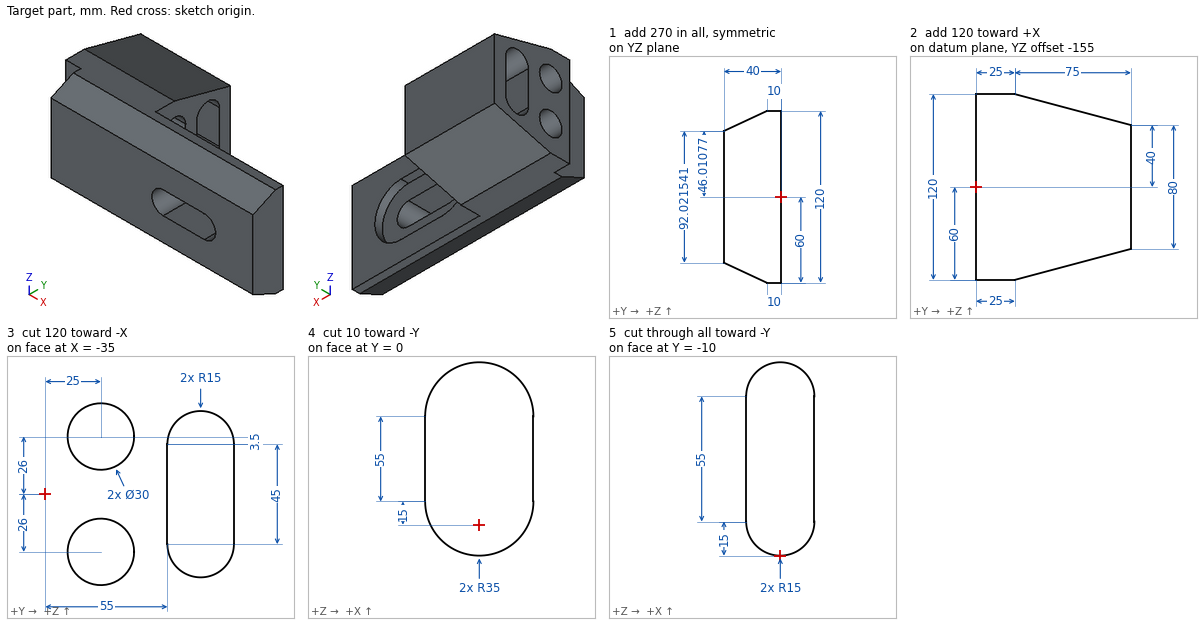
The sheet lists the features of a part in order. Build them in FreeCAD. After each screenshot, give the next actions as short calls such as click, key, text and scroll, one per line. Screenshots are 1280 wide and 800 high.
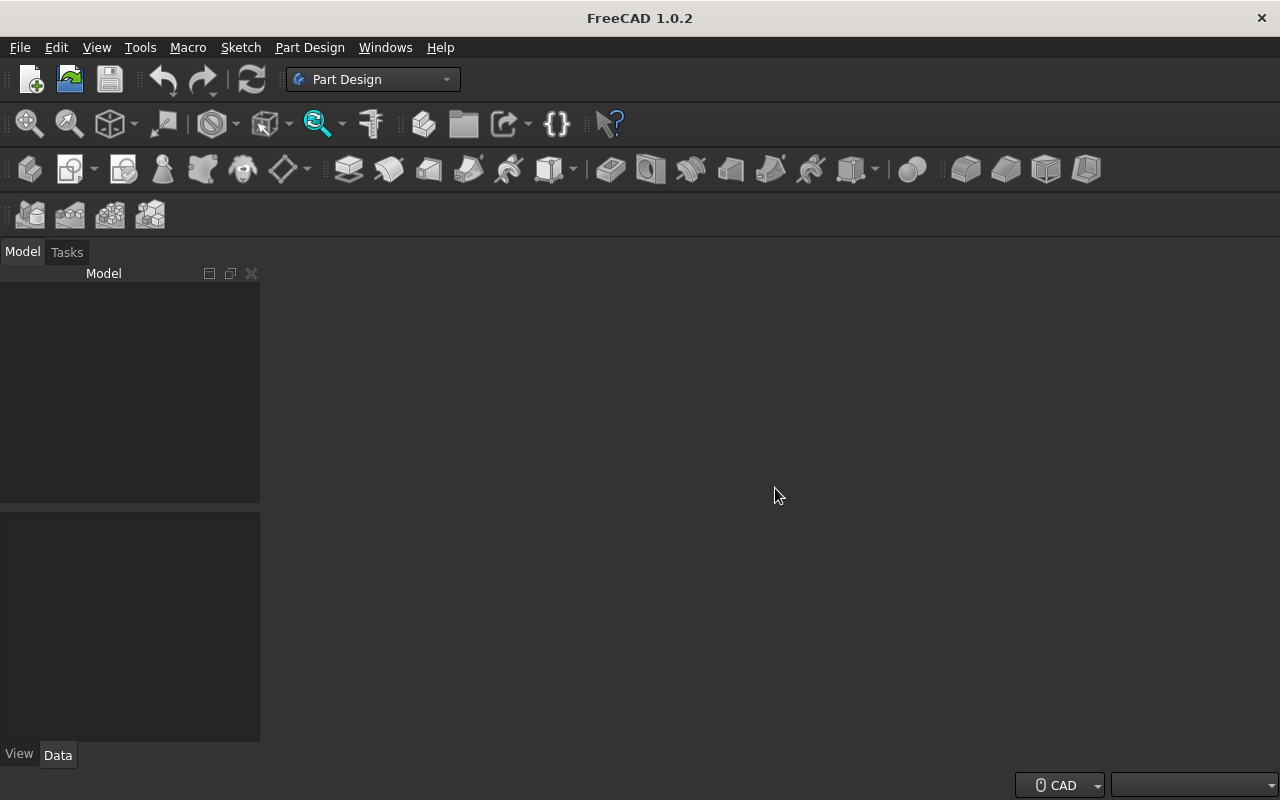
click(30, 80)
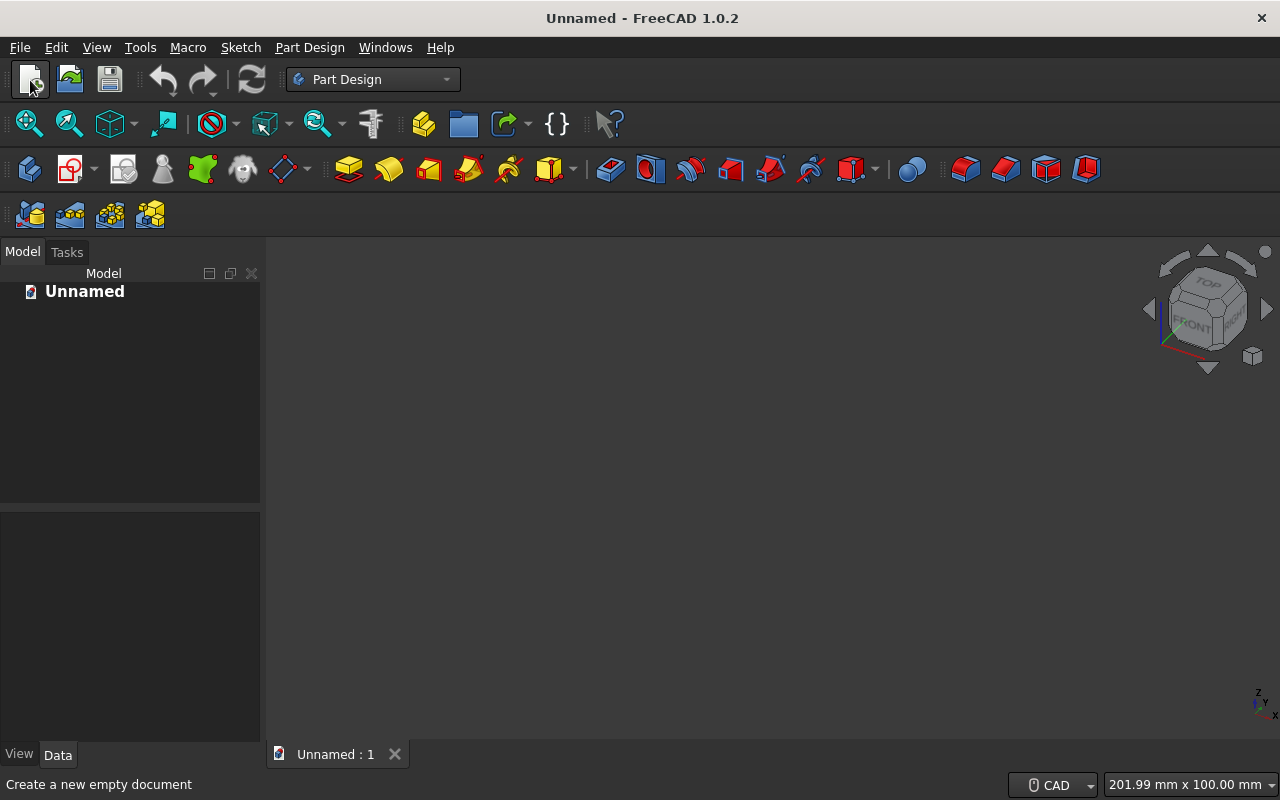
click(70, 170)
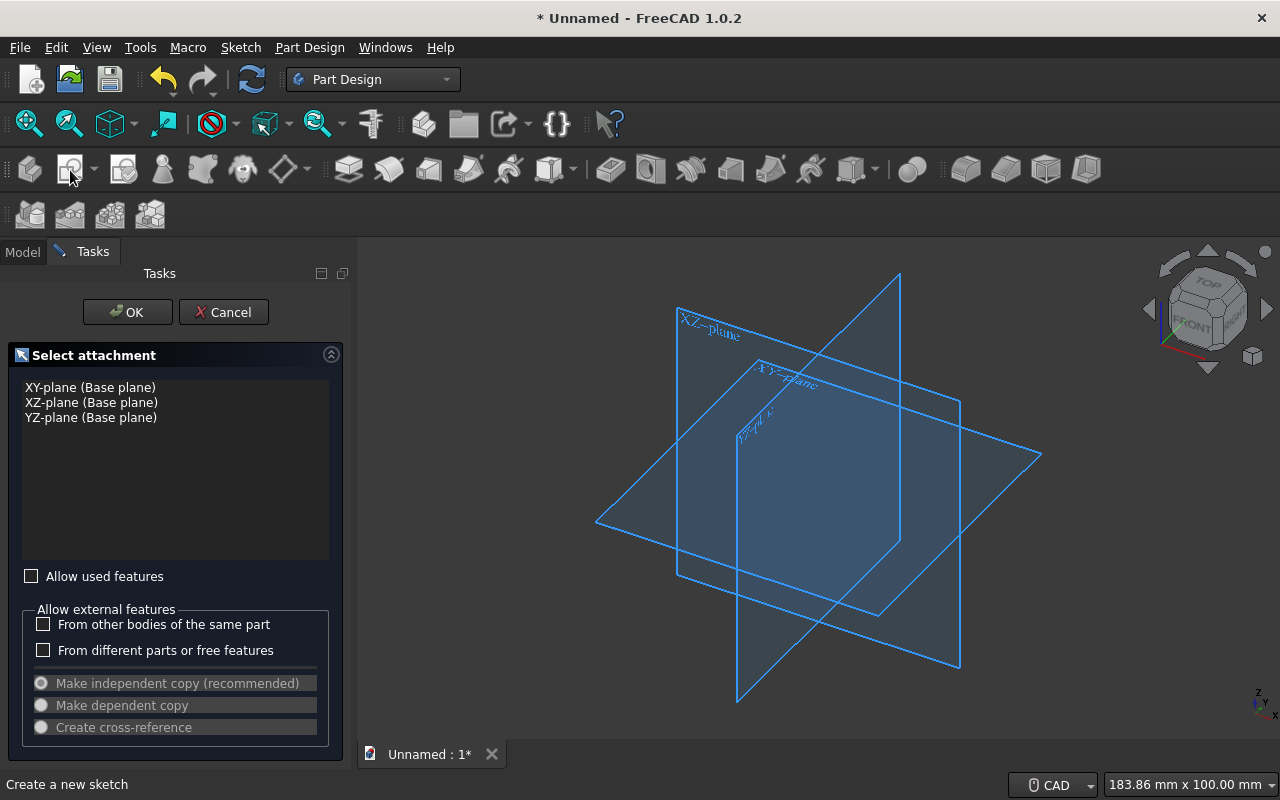
click(82, 418)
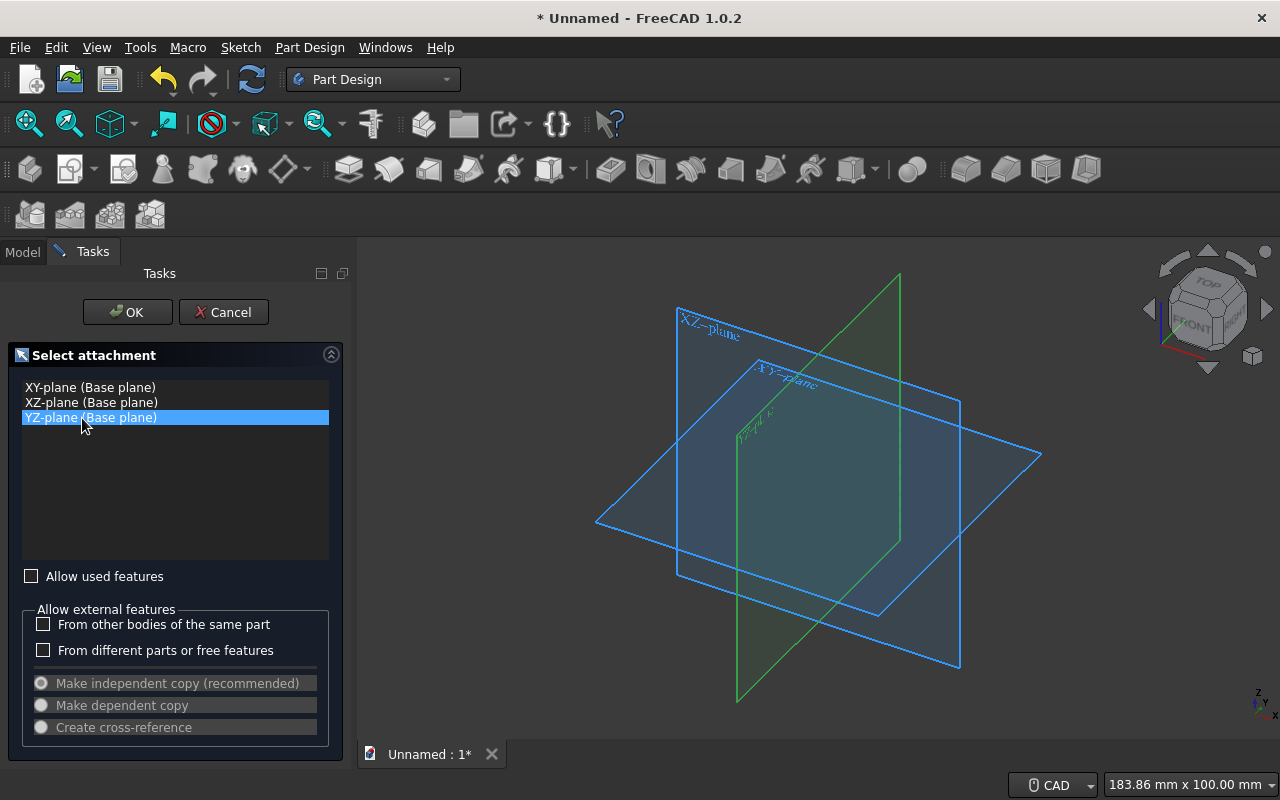
click(128, 312)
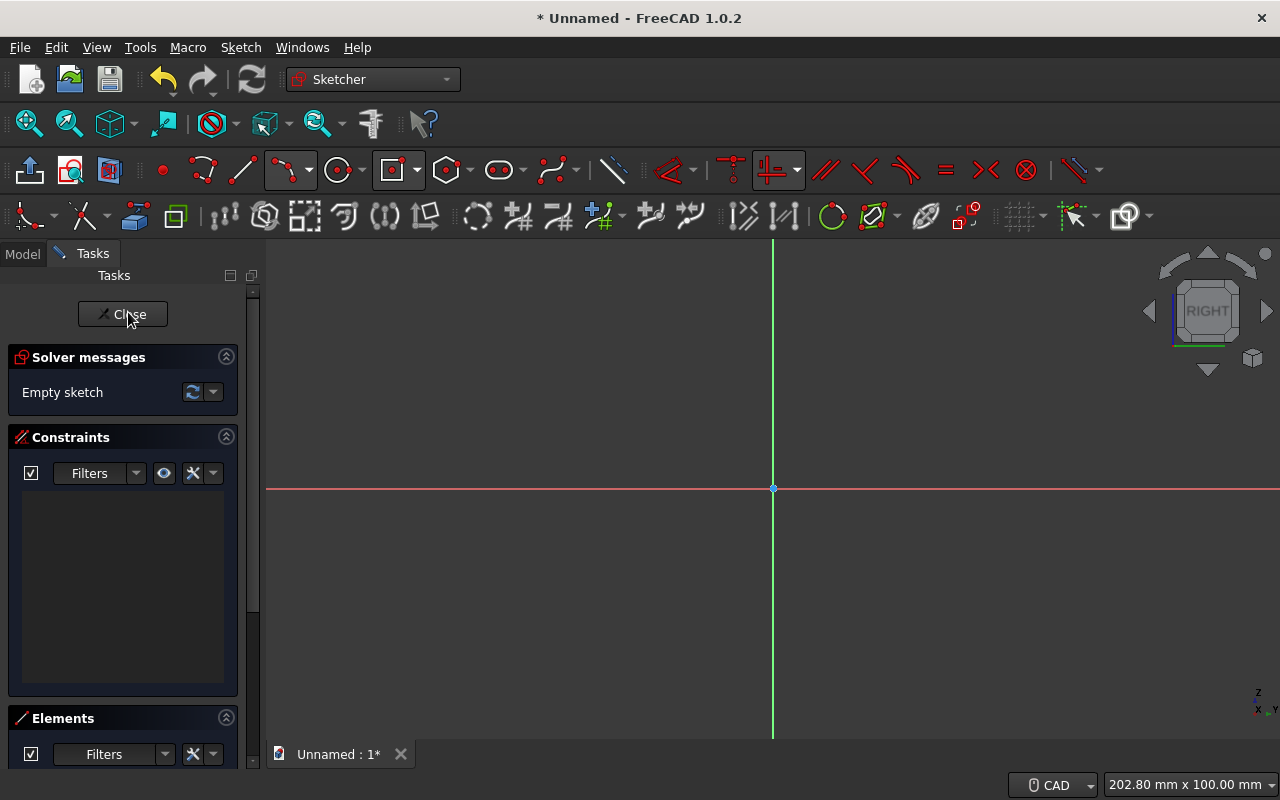
scroll(743, 489, down, 3)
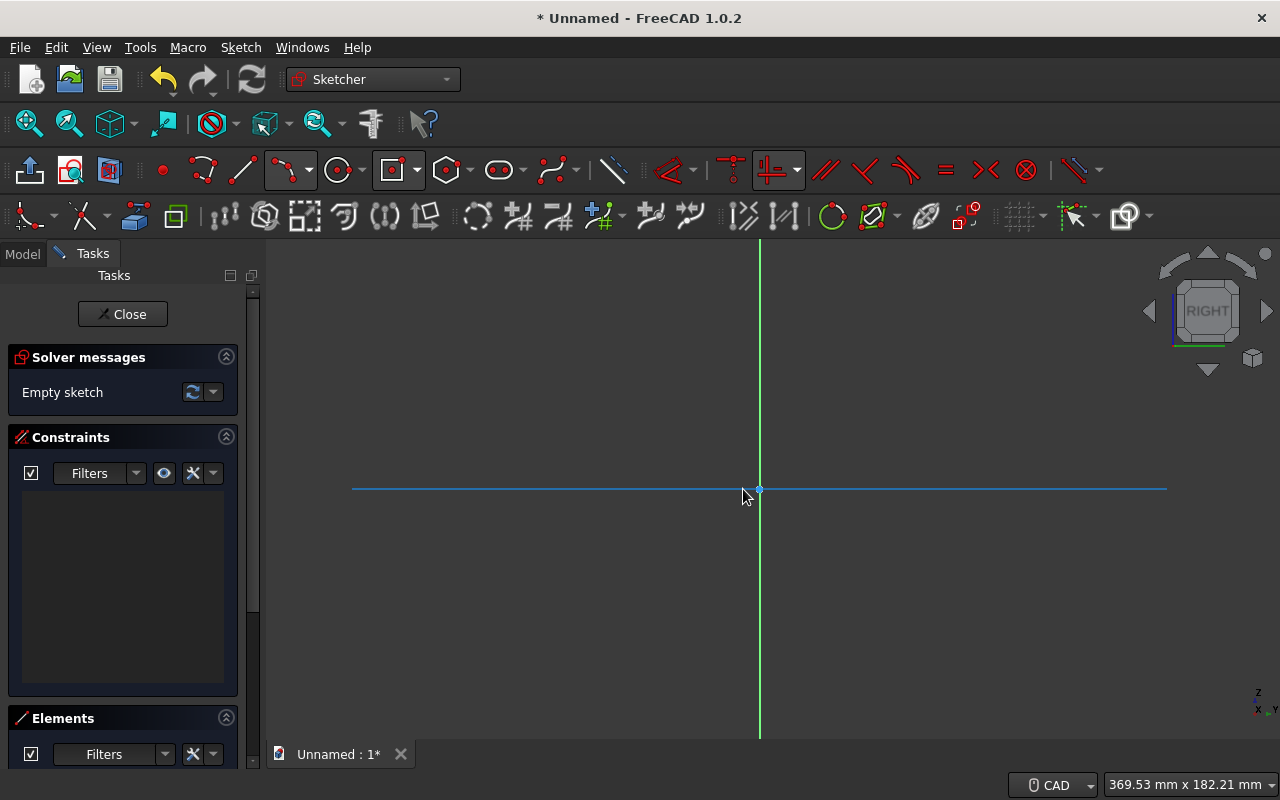
click(204, 170)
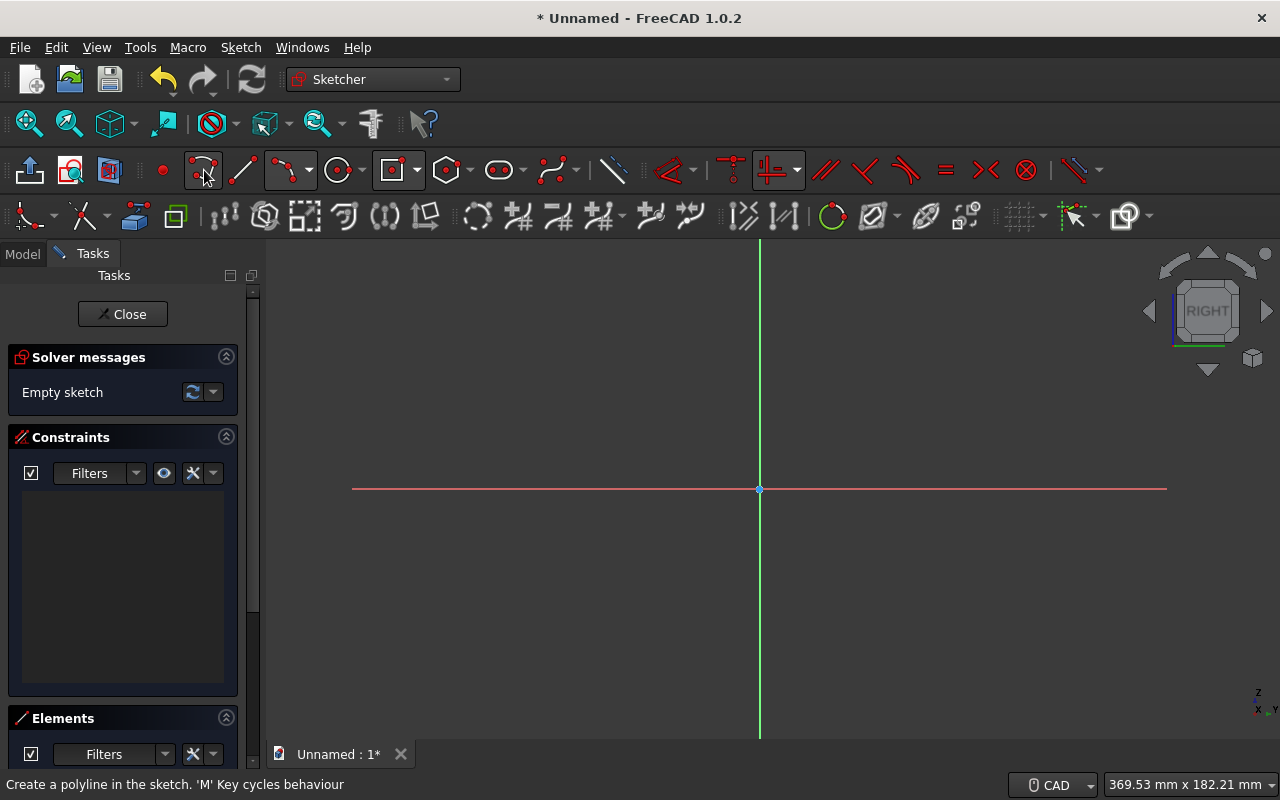
click(760, 654)
click(751, 325)
click(732, 325)
click(650, 363)
click(650, 615)
click(732, 654)
click(760, 655)
key(Escape)
key(Escape)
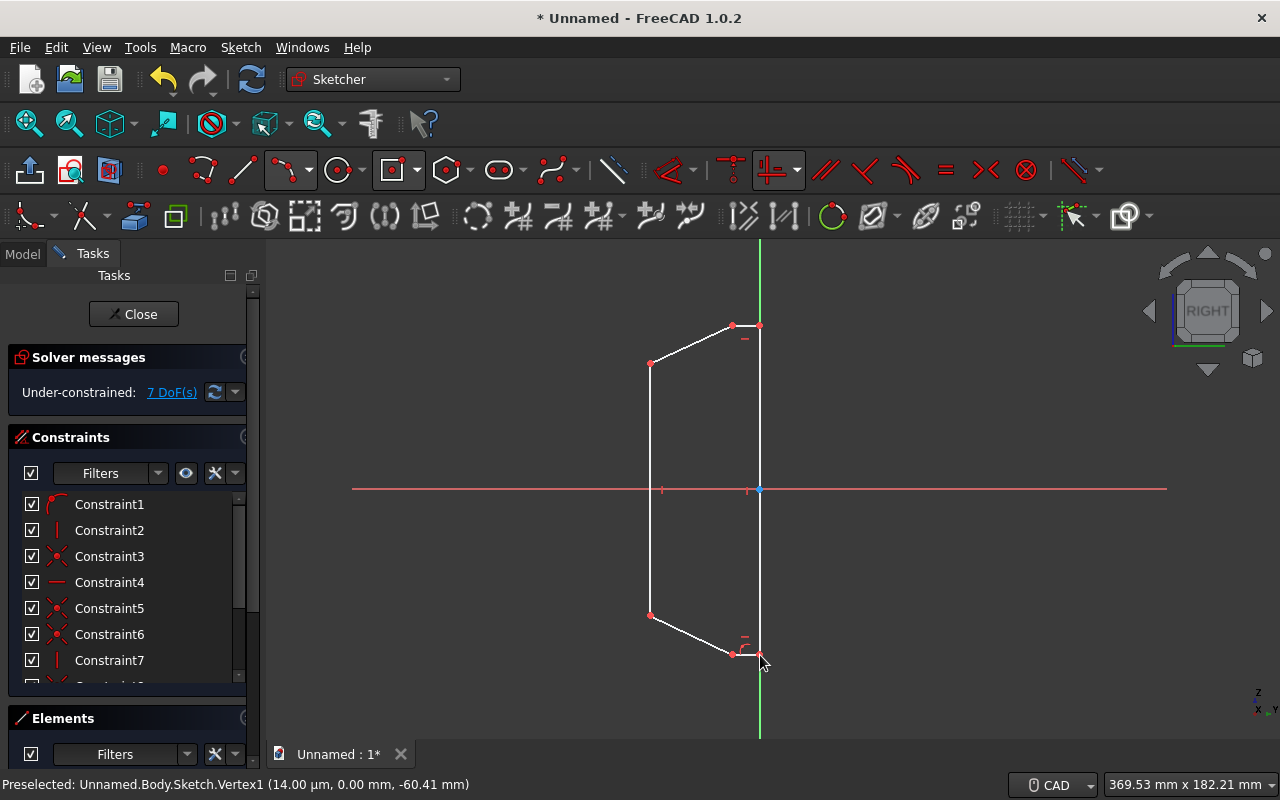
click(668, 170)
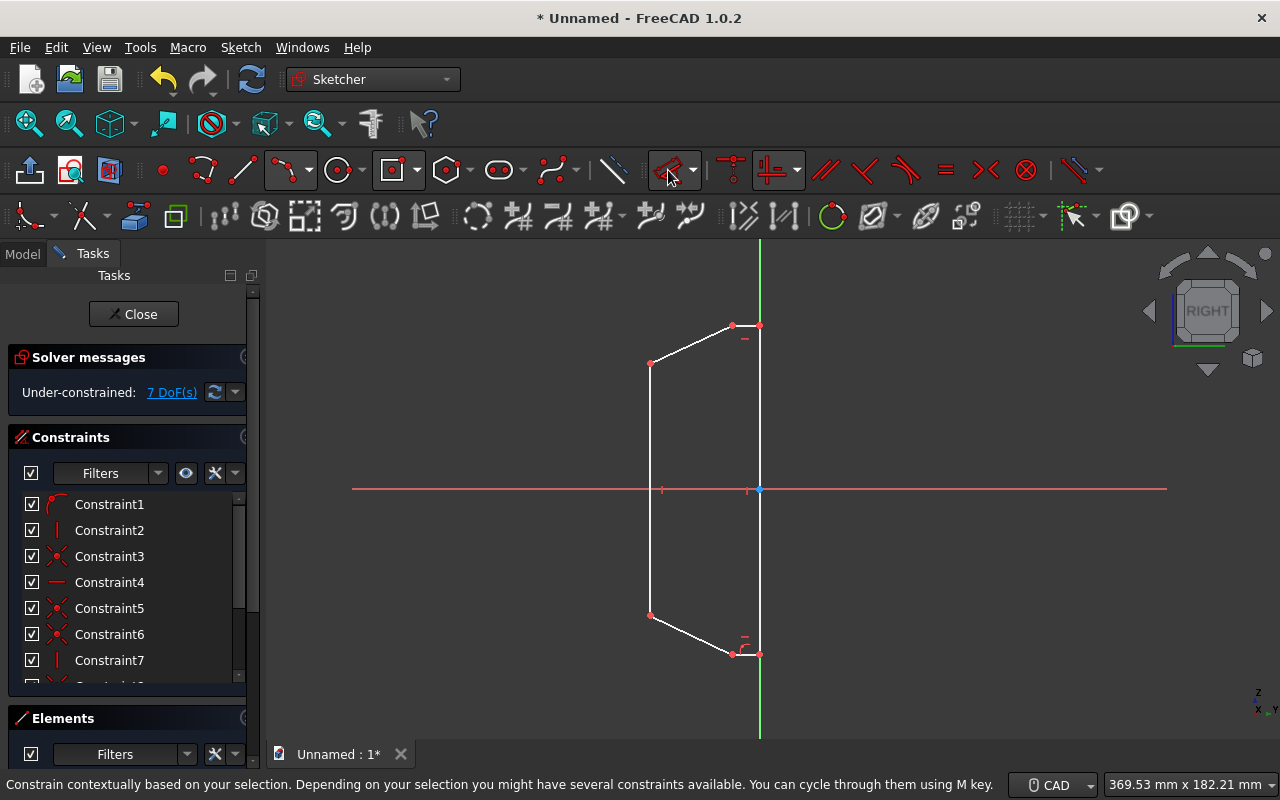
scroll(749, 326, up, 2)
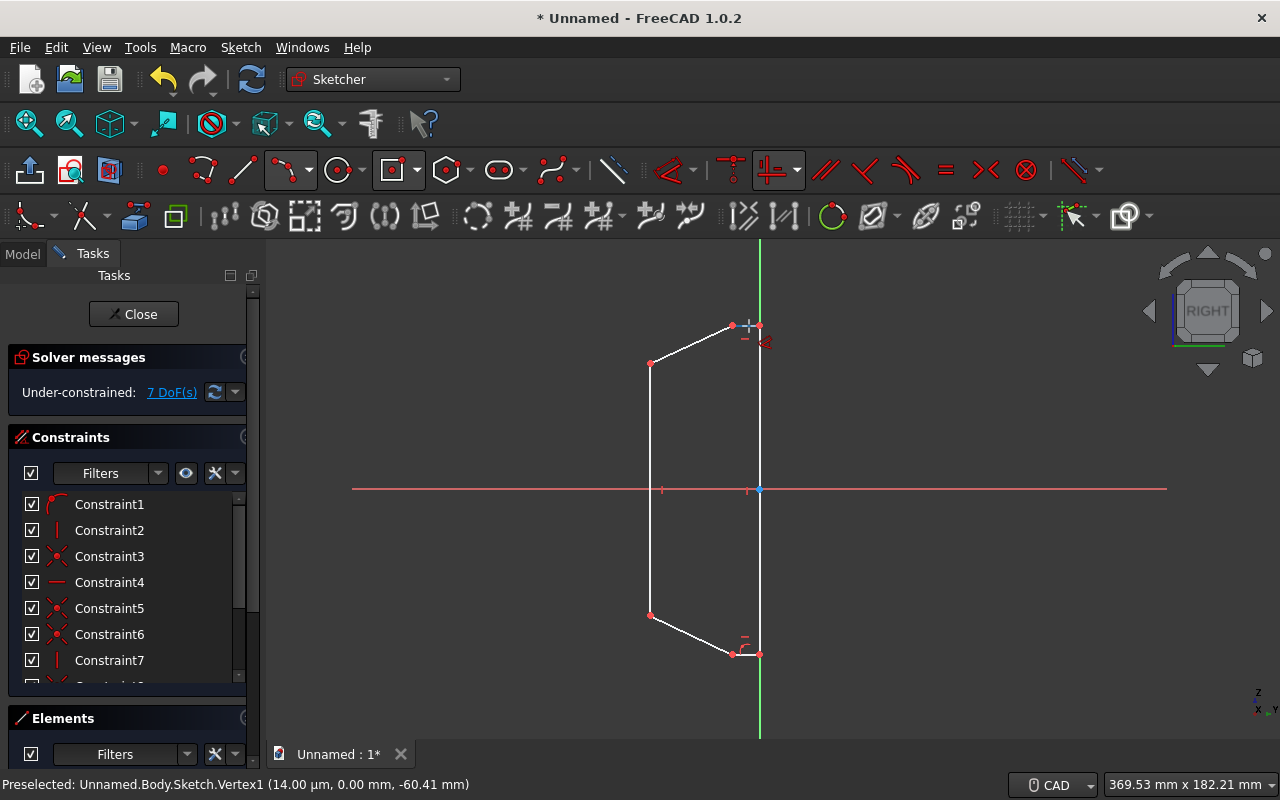
click(748, 326)
click(744, 292)